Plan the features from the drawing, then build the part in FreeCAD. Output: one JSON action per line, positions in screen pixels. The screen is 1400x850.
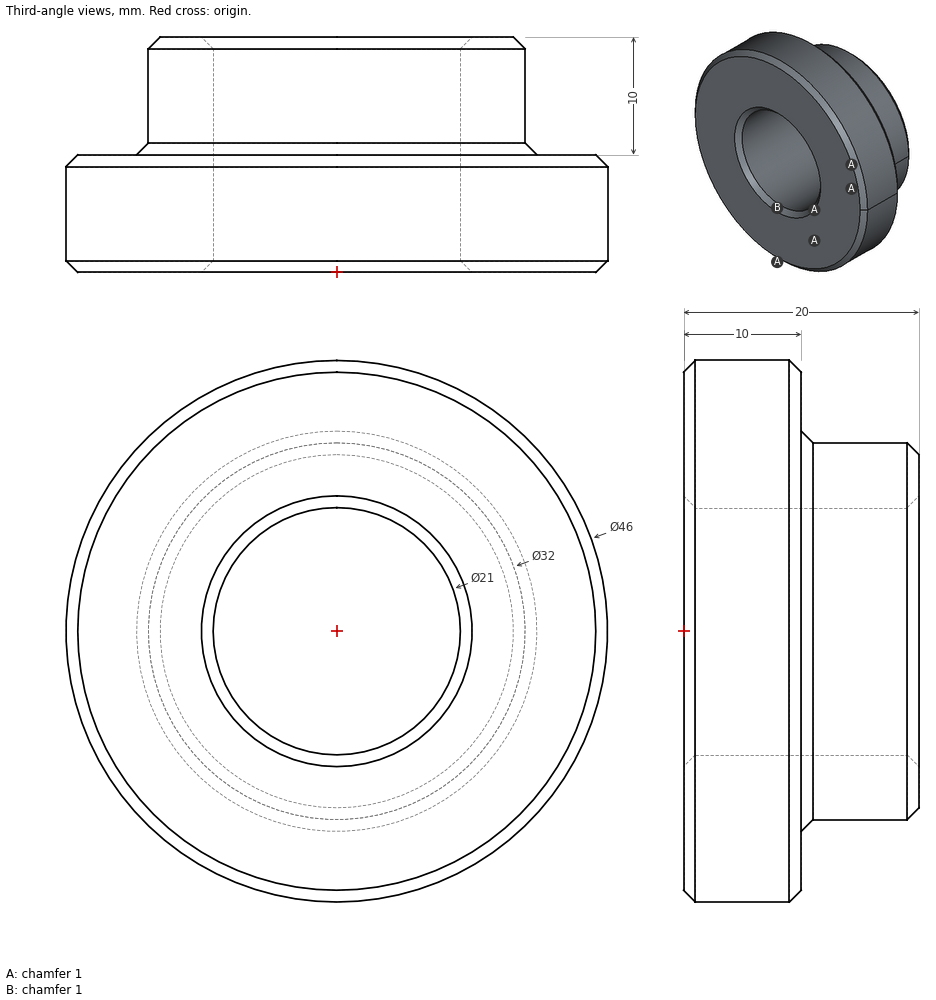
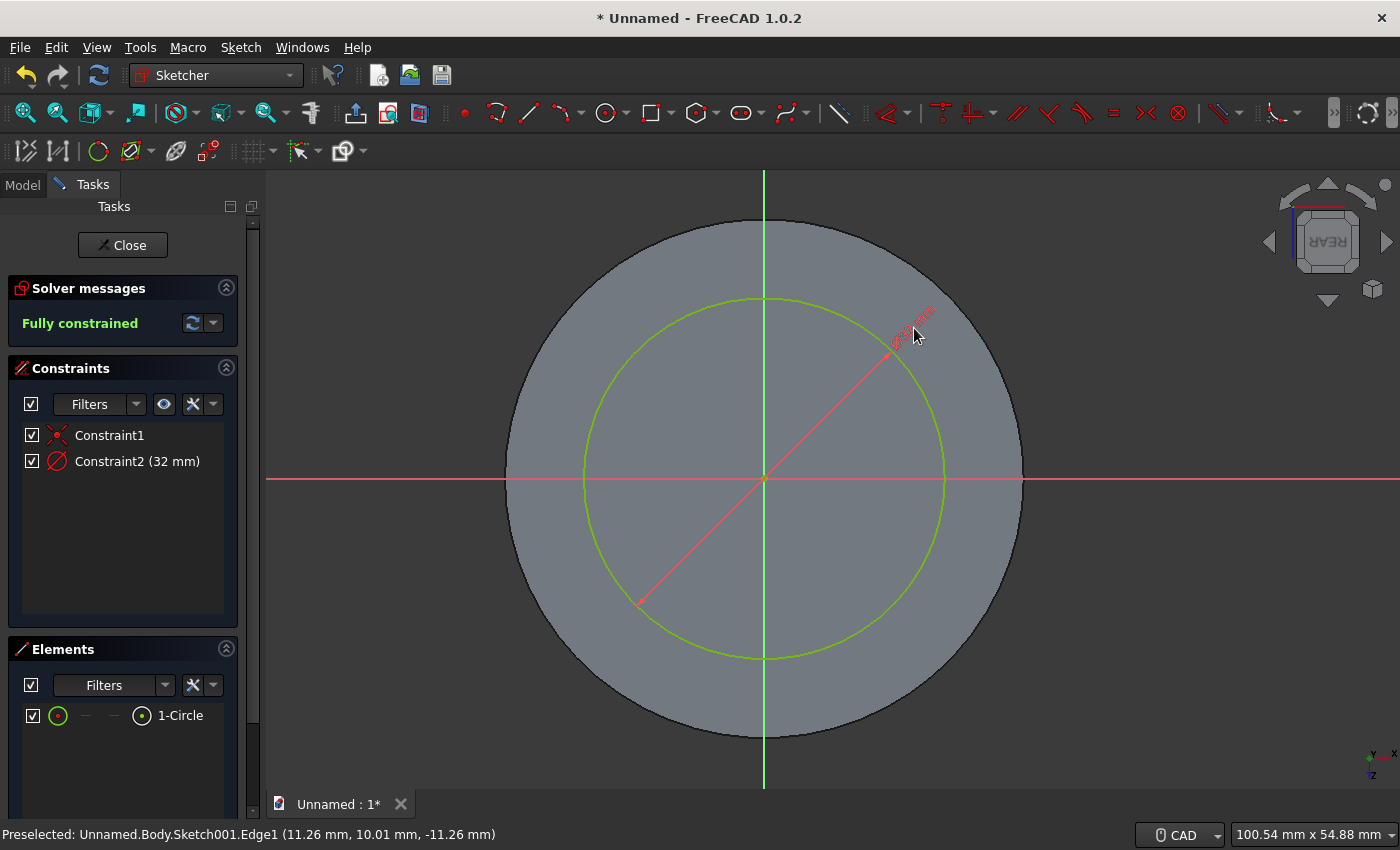
{"action": "left_click", "coordinate": [123, 245]}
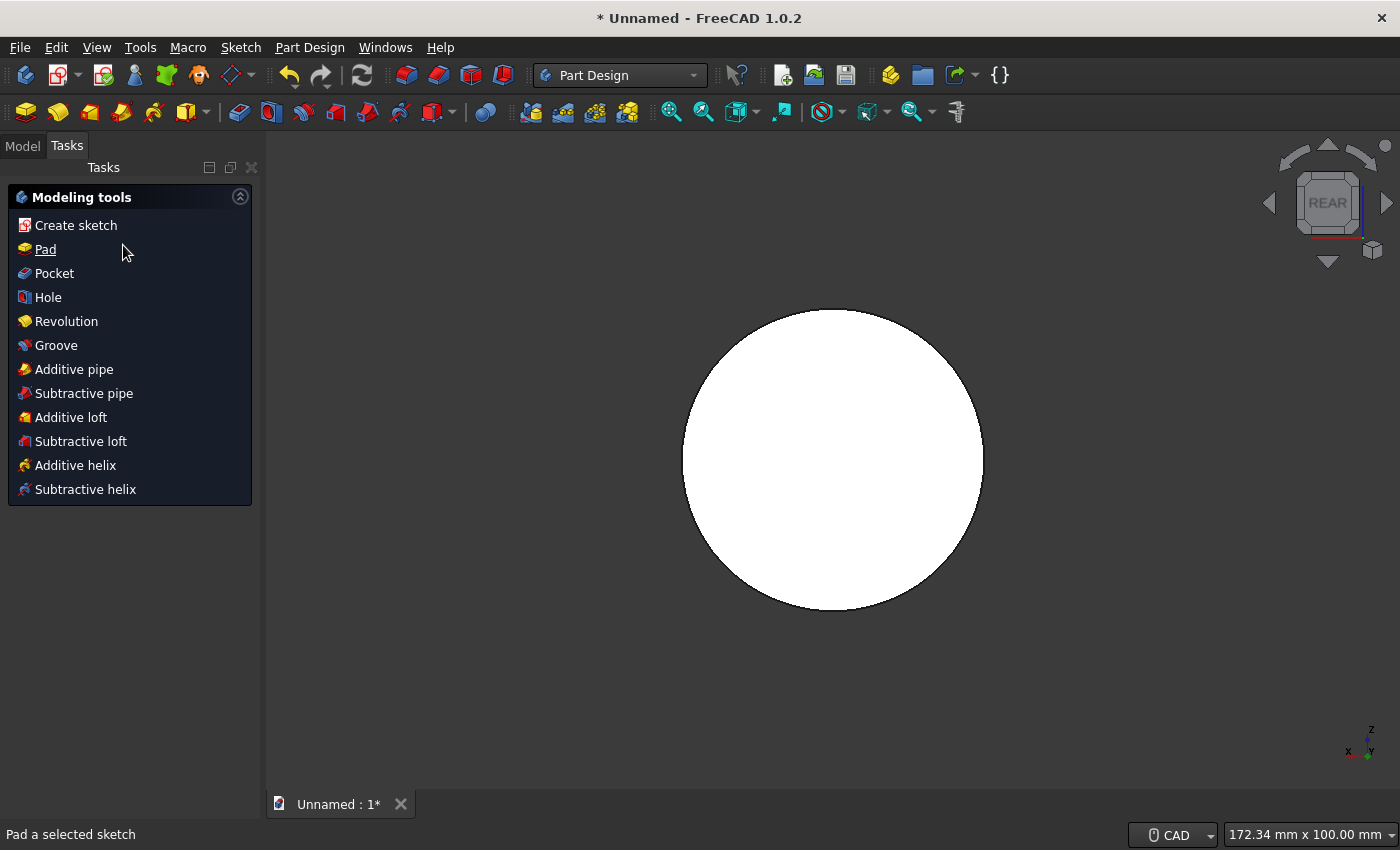
{"action": "left_click", "coordinate": [26, 112]}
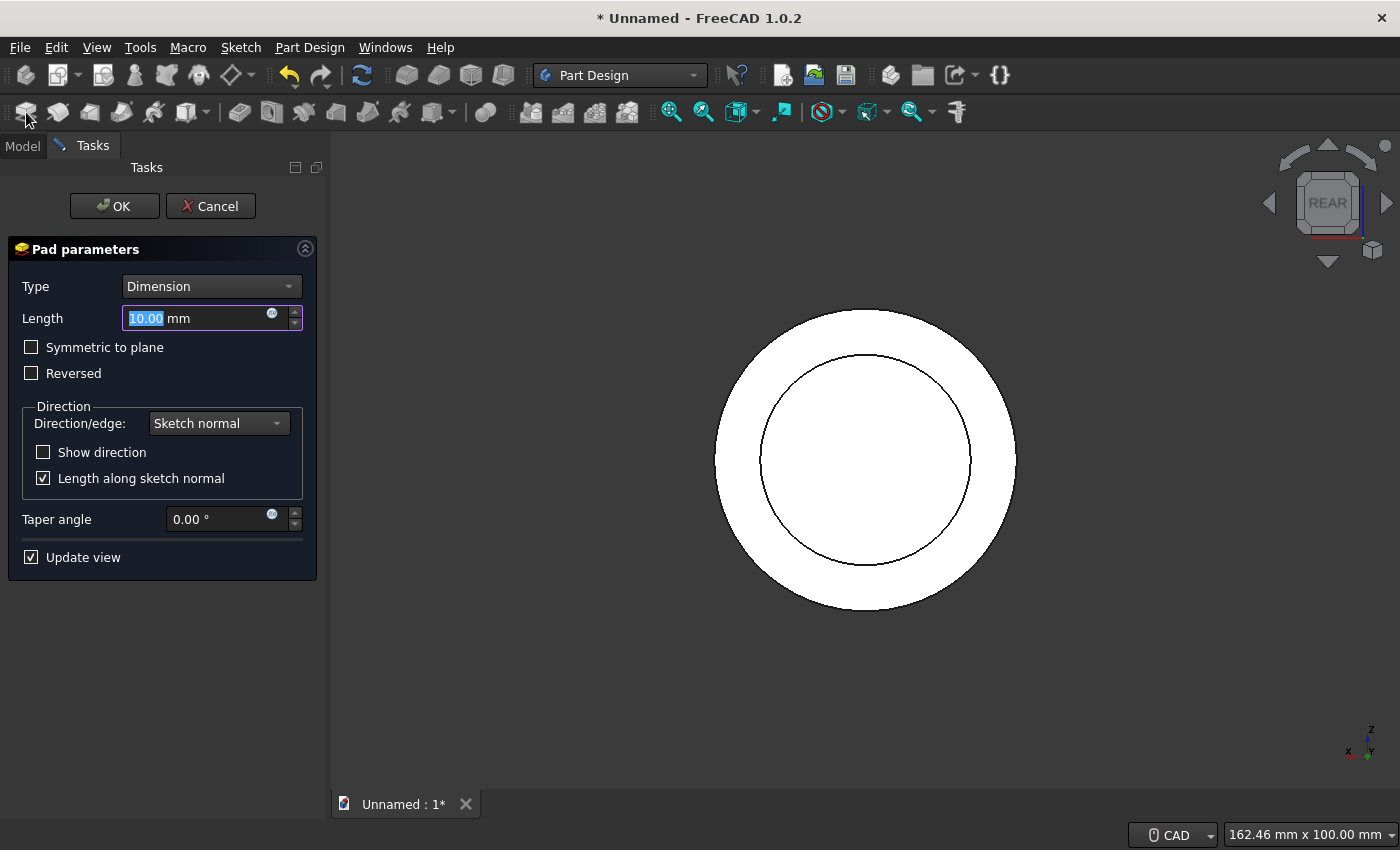
{"action": "type", "text": "10"}
{"action": "key", "text": "Tab"}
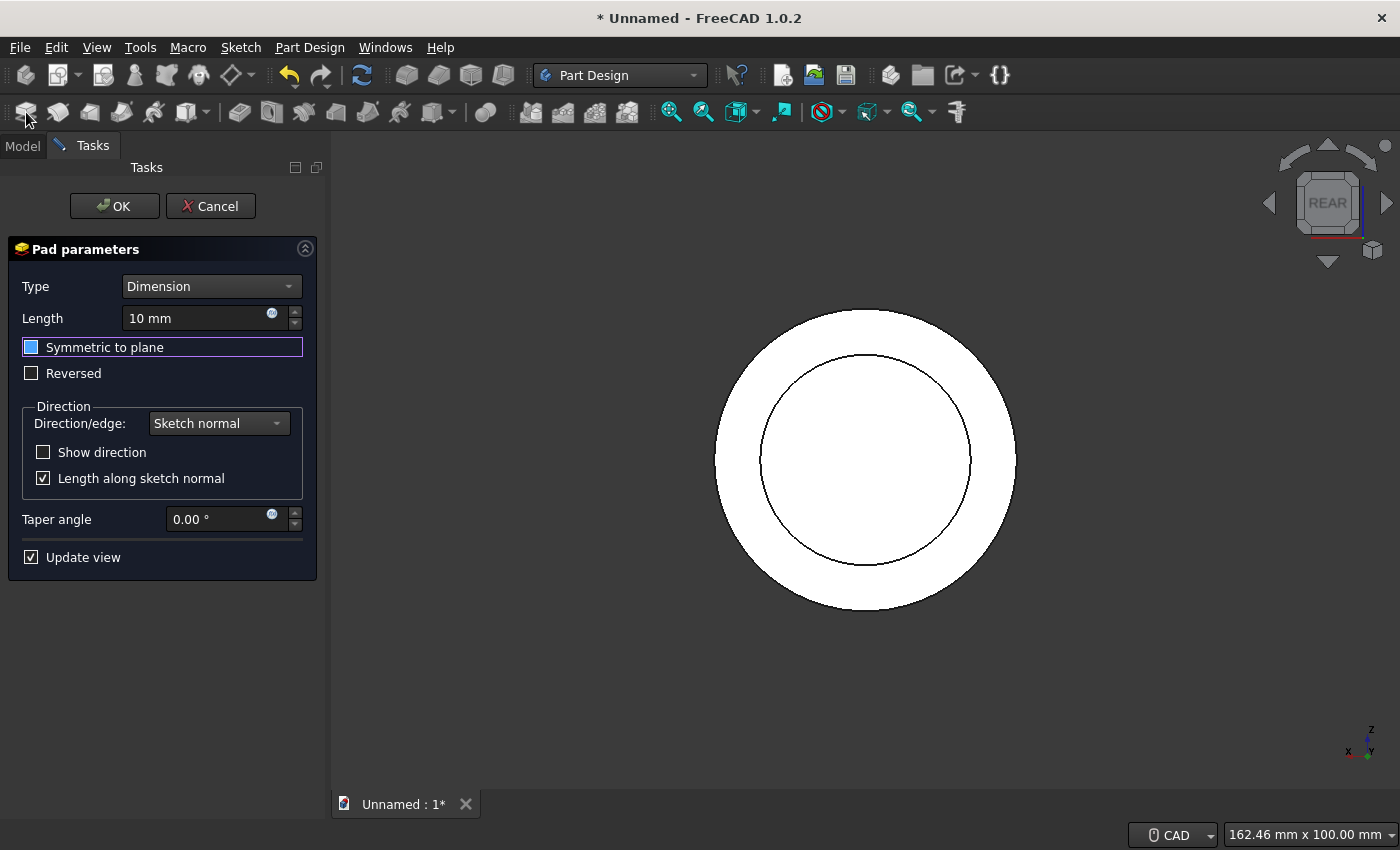
{"action": "left_click", "coordinate": [115, 206]}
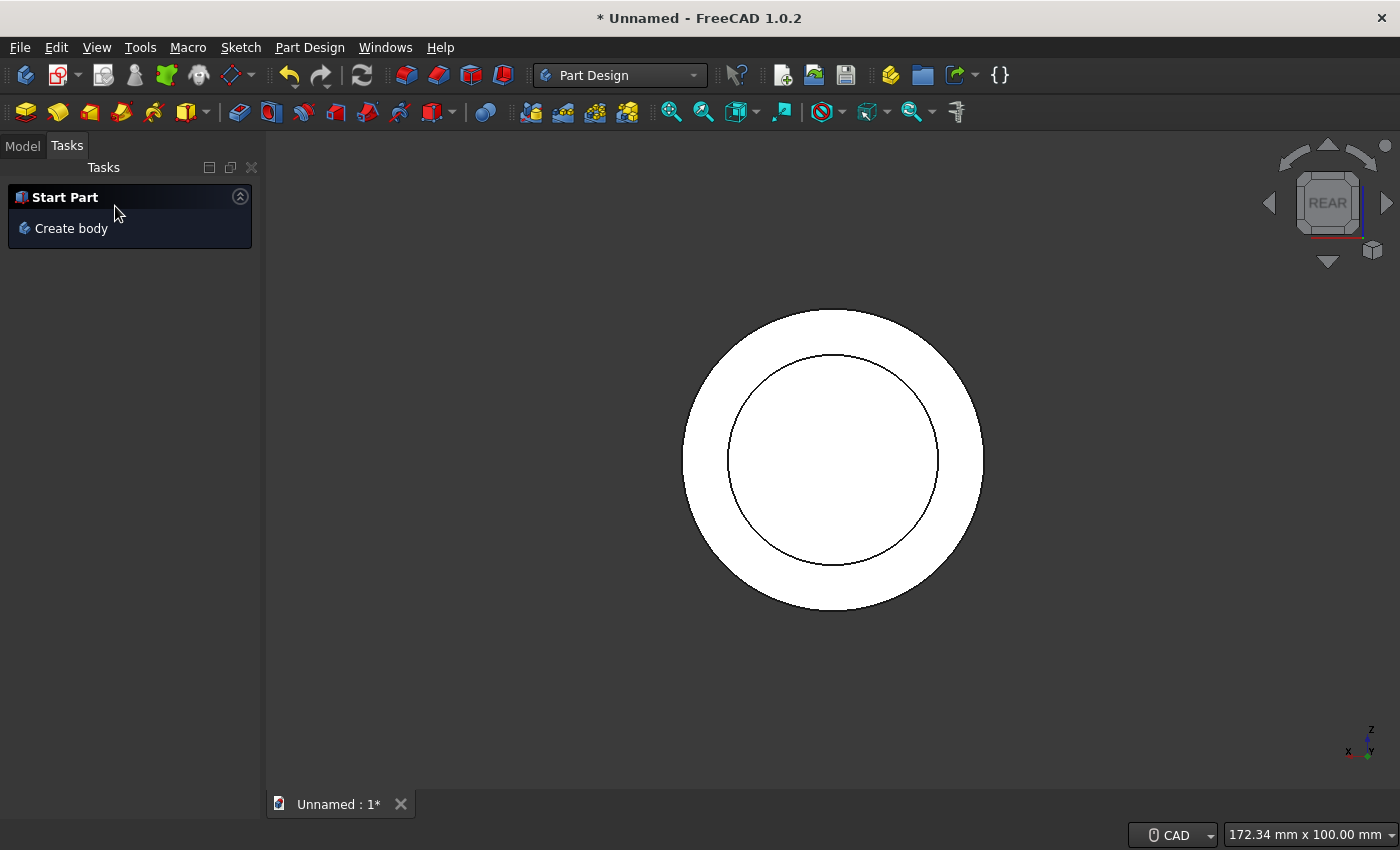
{"action": "left_click", "coordinate": [833, 459]}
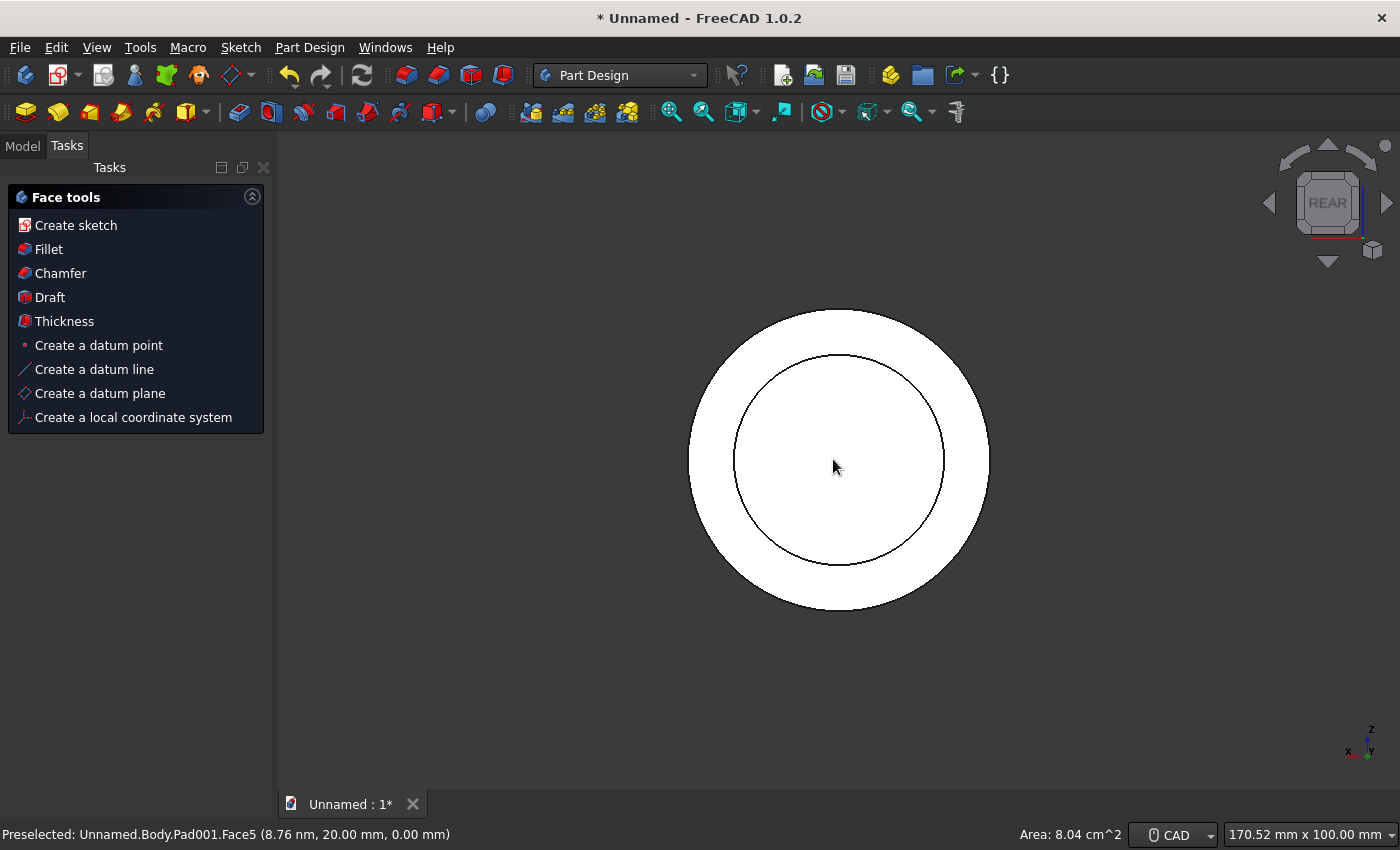
{"action": "left_click", "coordinate": [58, 76]}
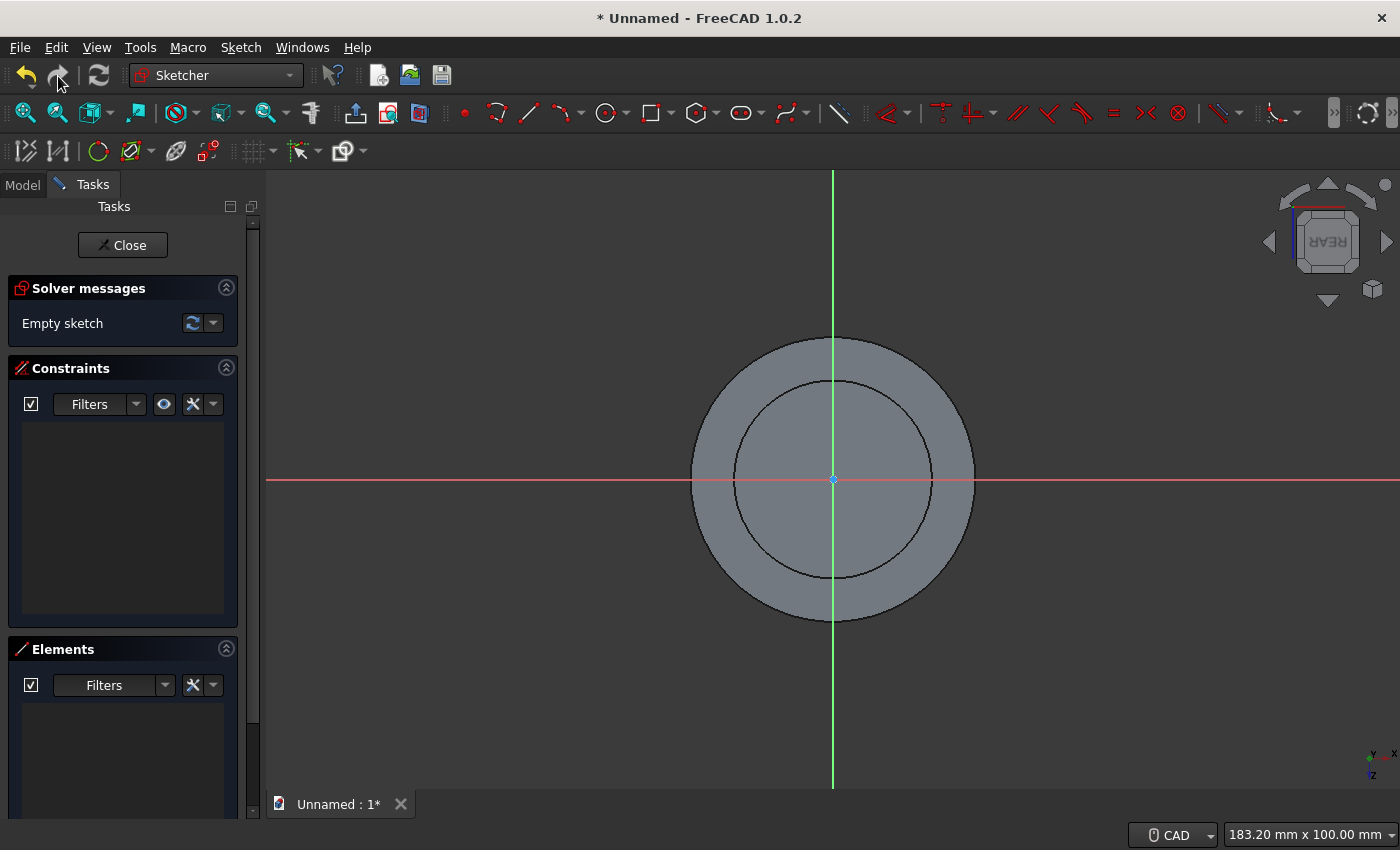
{"action": "scroll", "coordinate": [863, 479], "scroll_direction": "up", "scroll_amount": 6}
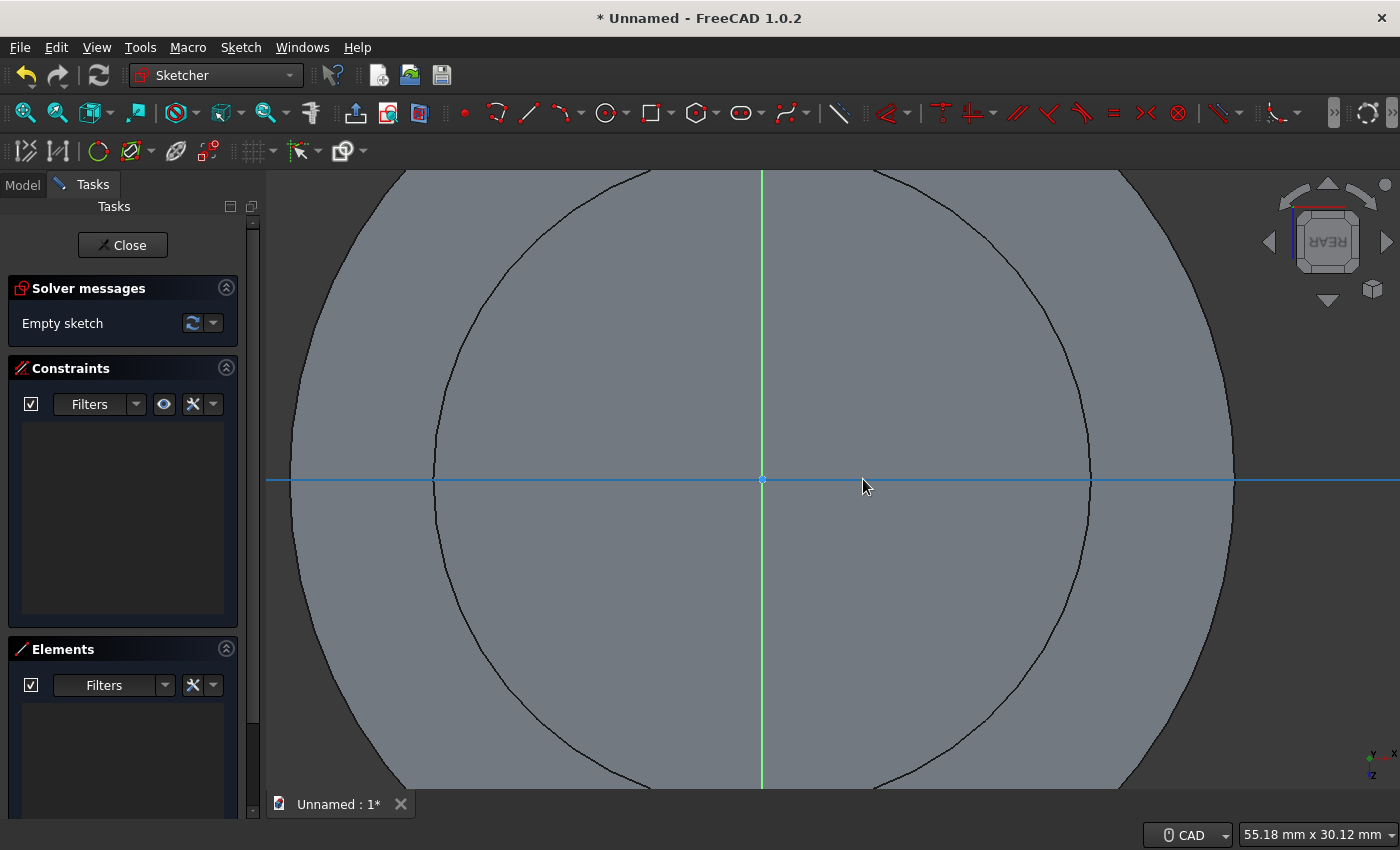
{"action": "key", "text": "g c"}